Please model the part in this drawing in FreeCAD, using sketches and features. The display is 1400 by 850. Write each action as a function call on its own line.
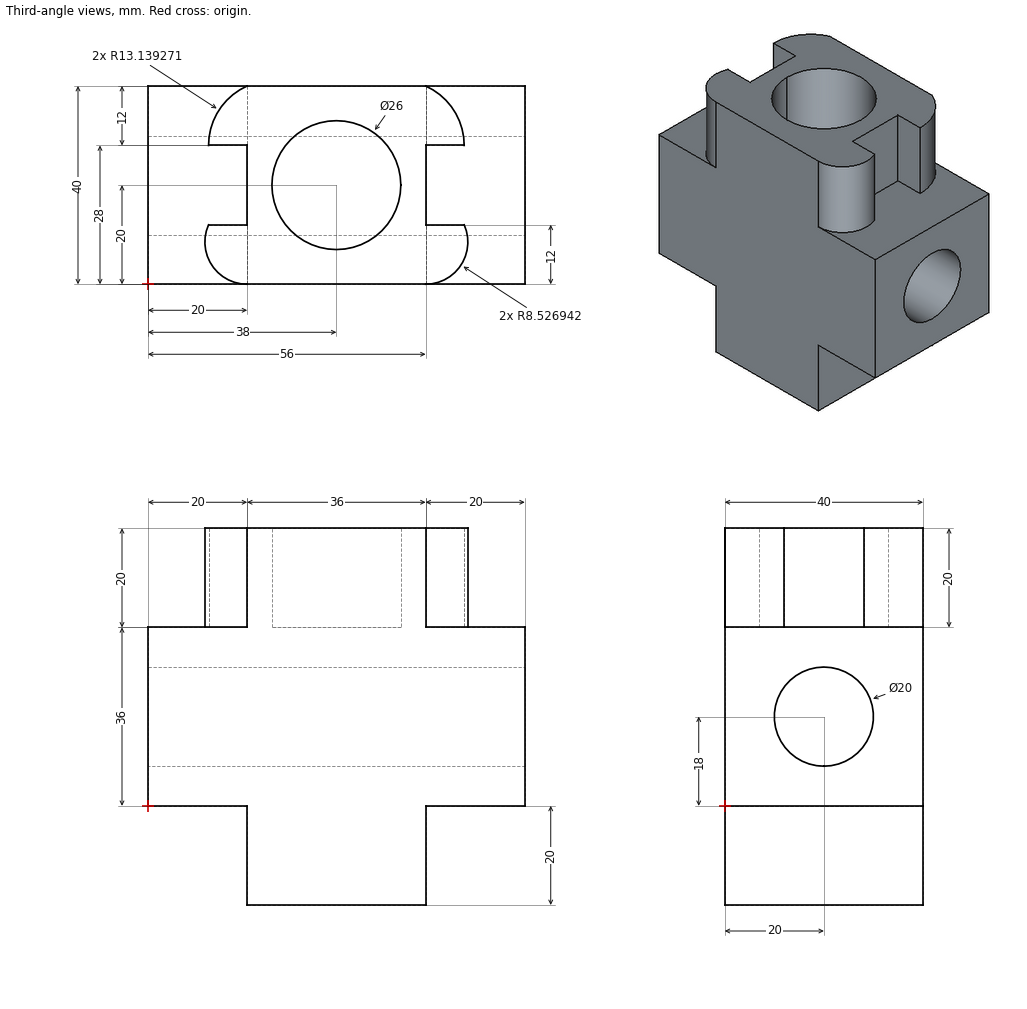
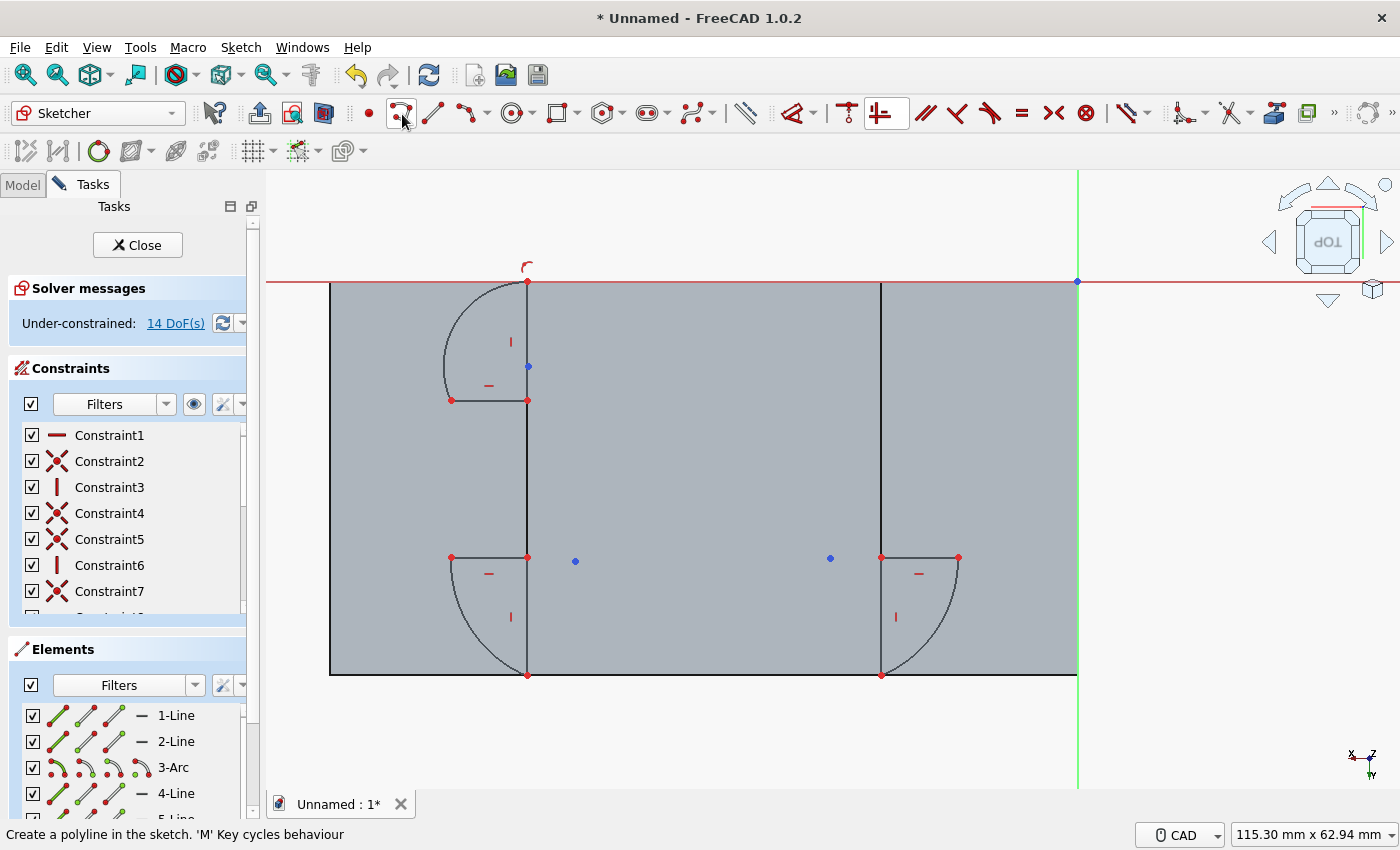
click(881, 282)
click(881, 400)
click(958, 400)
right_click(958, 400)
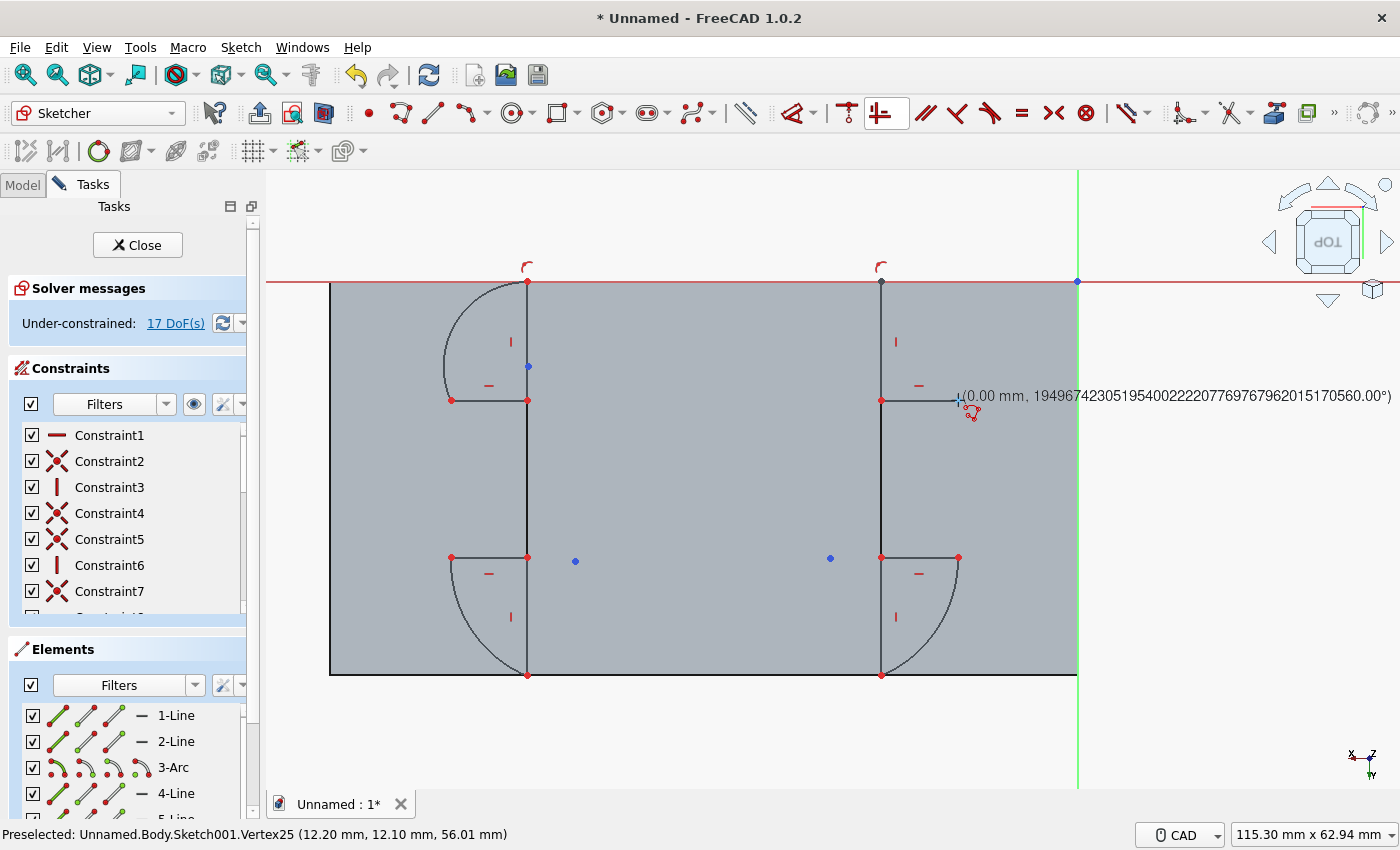
click(466, 114)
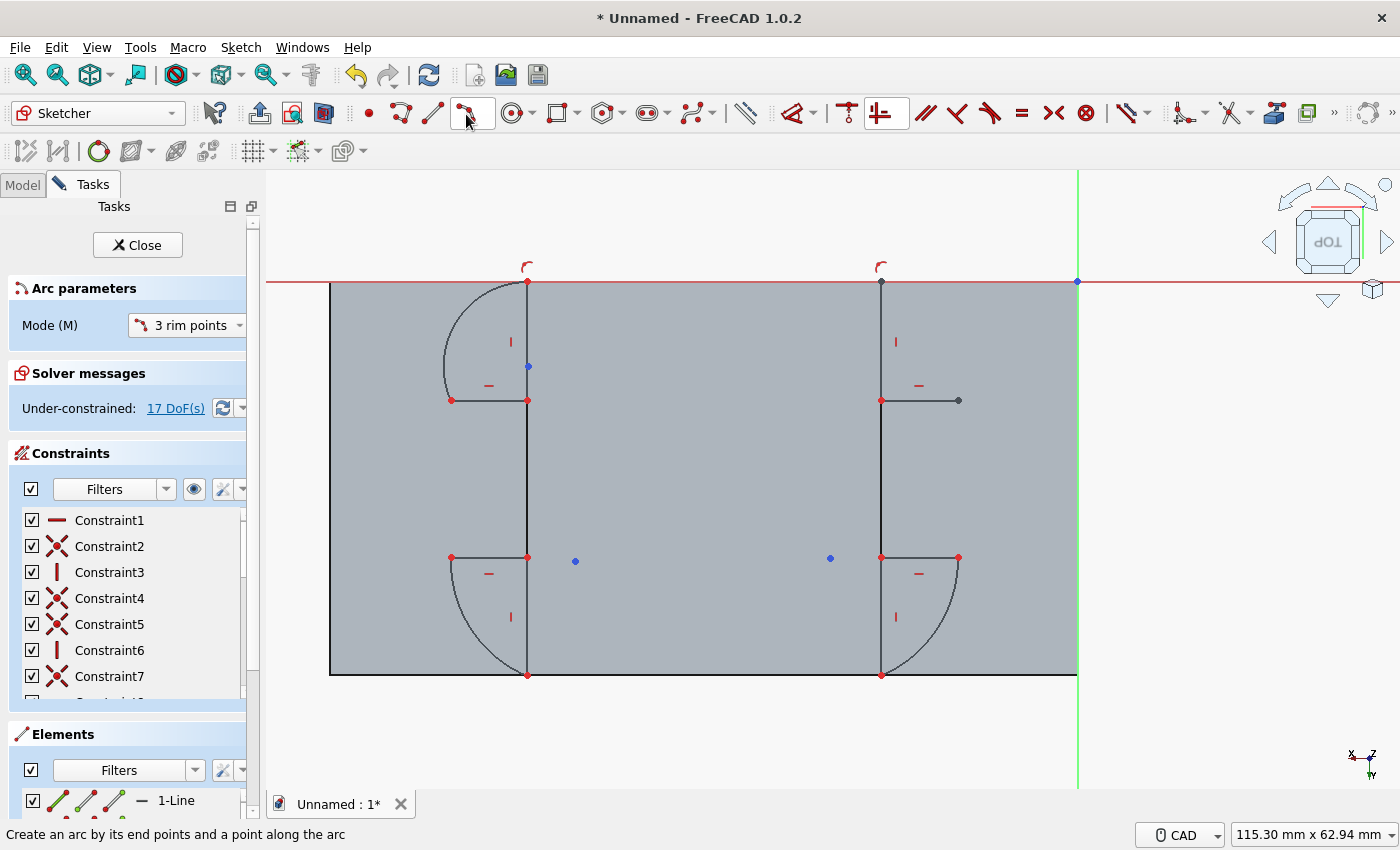
click(958, 401)
click(881, 282)
click(952, 320)
key(Escape)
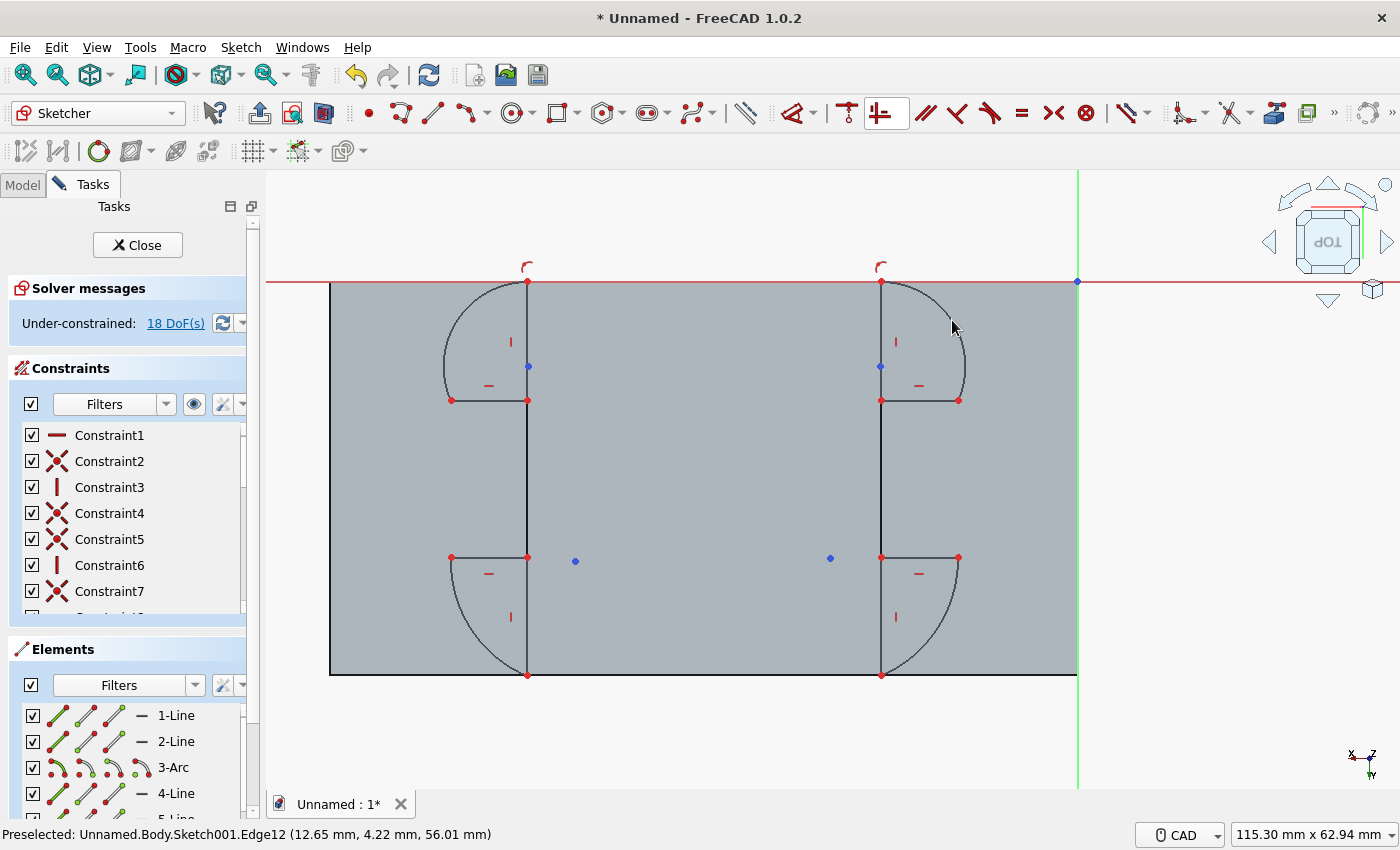
click(918, 651)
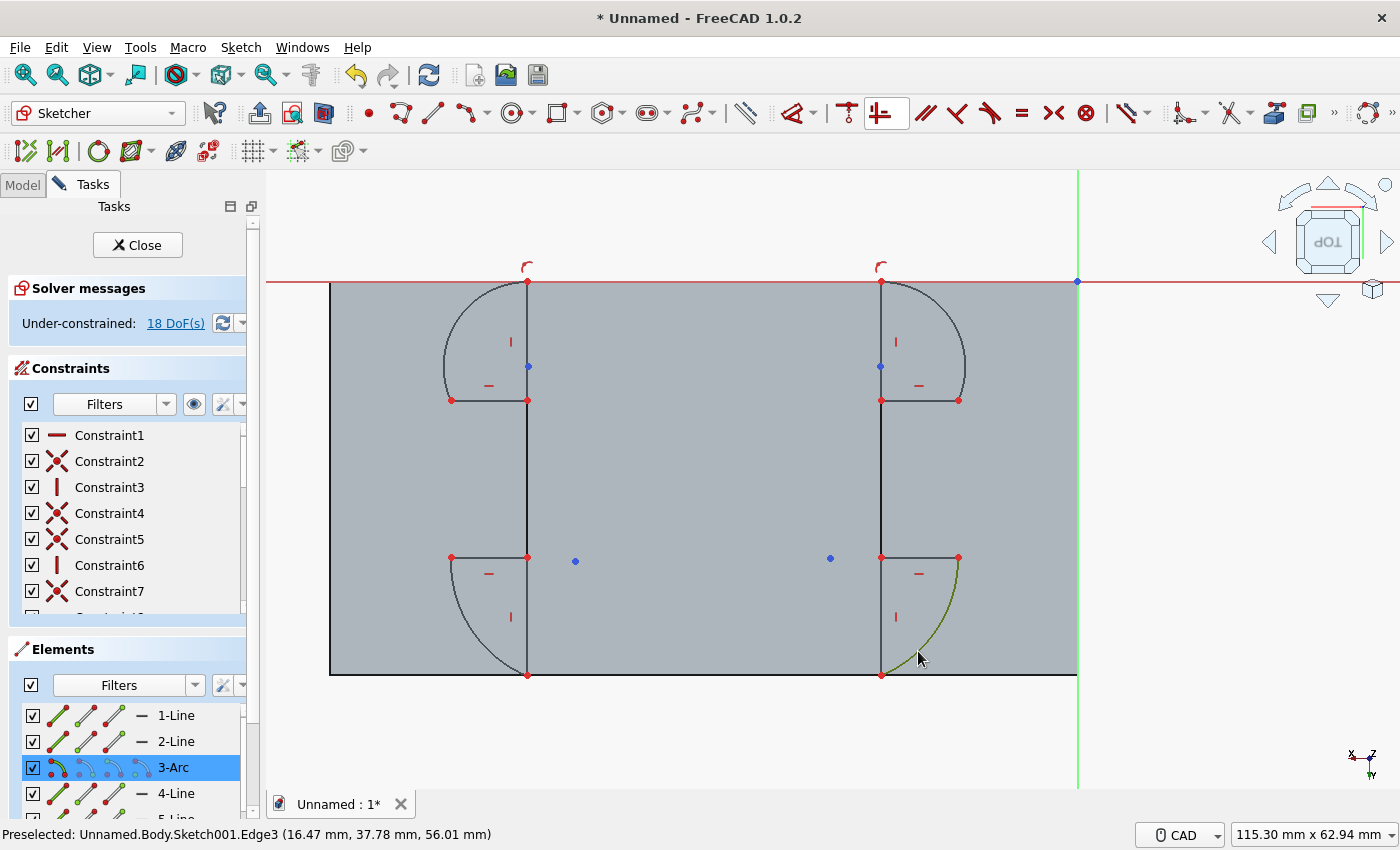
click(458, 602)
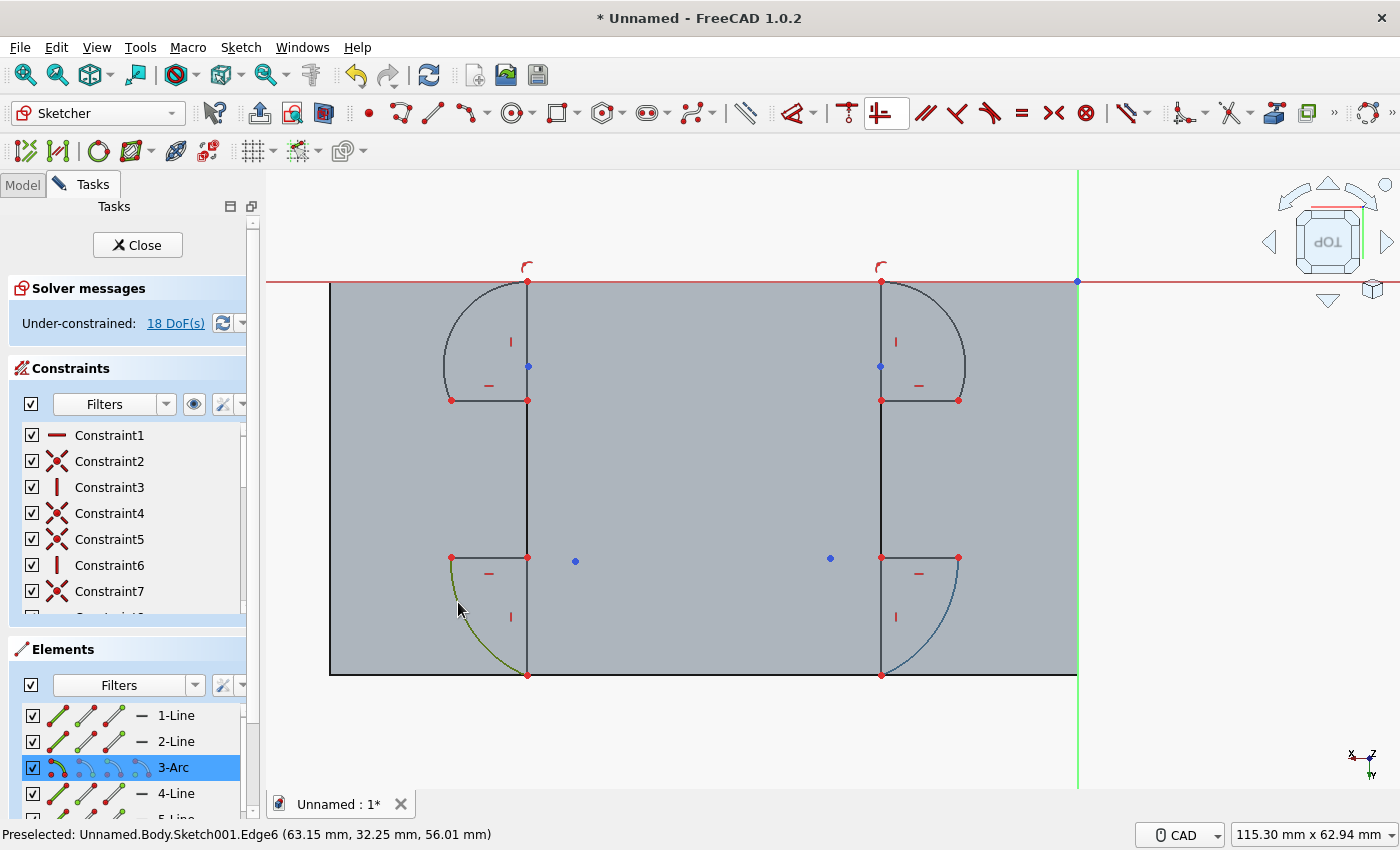
click(1022, 114)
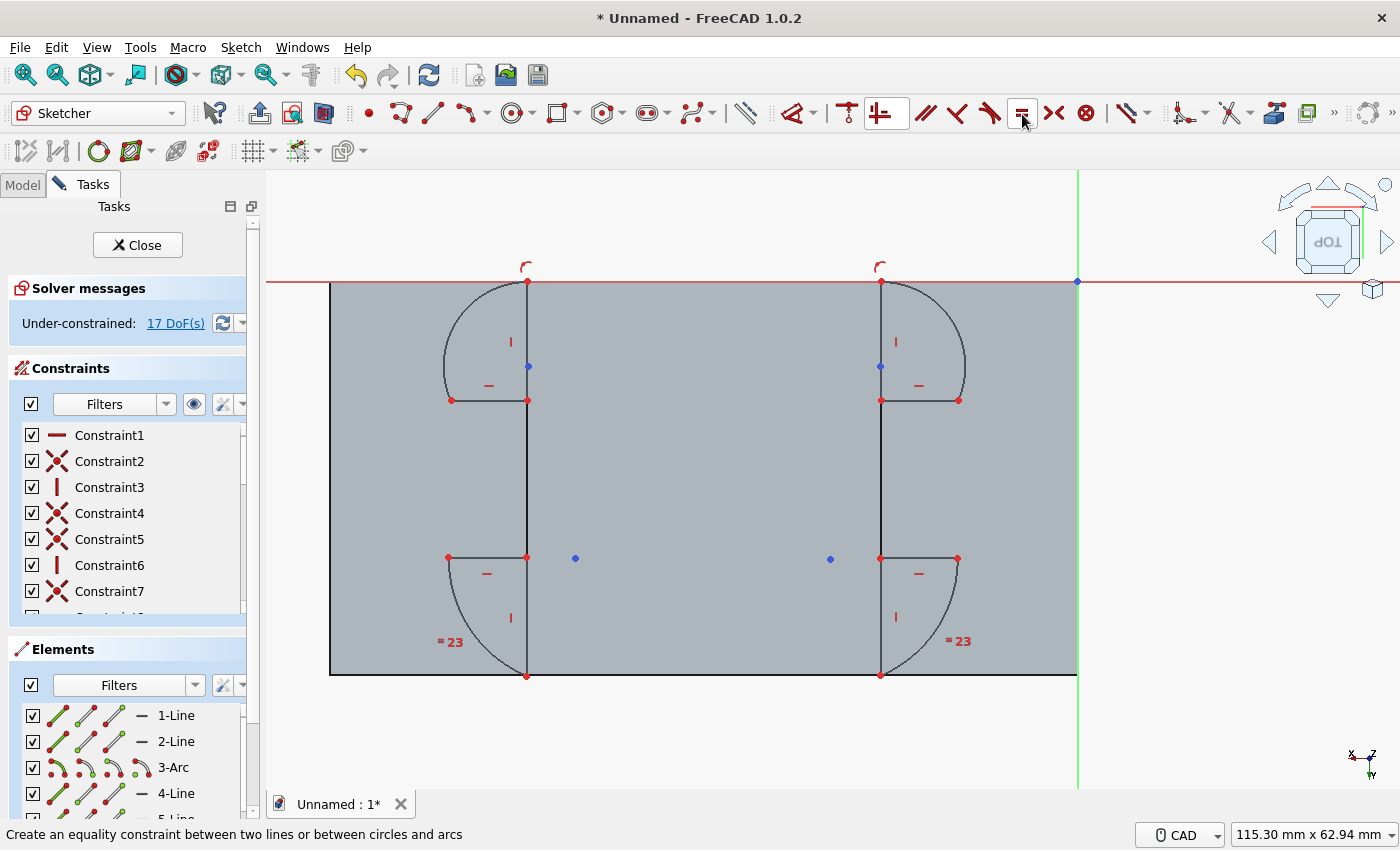
click(480, 297)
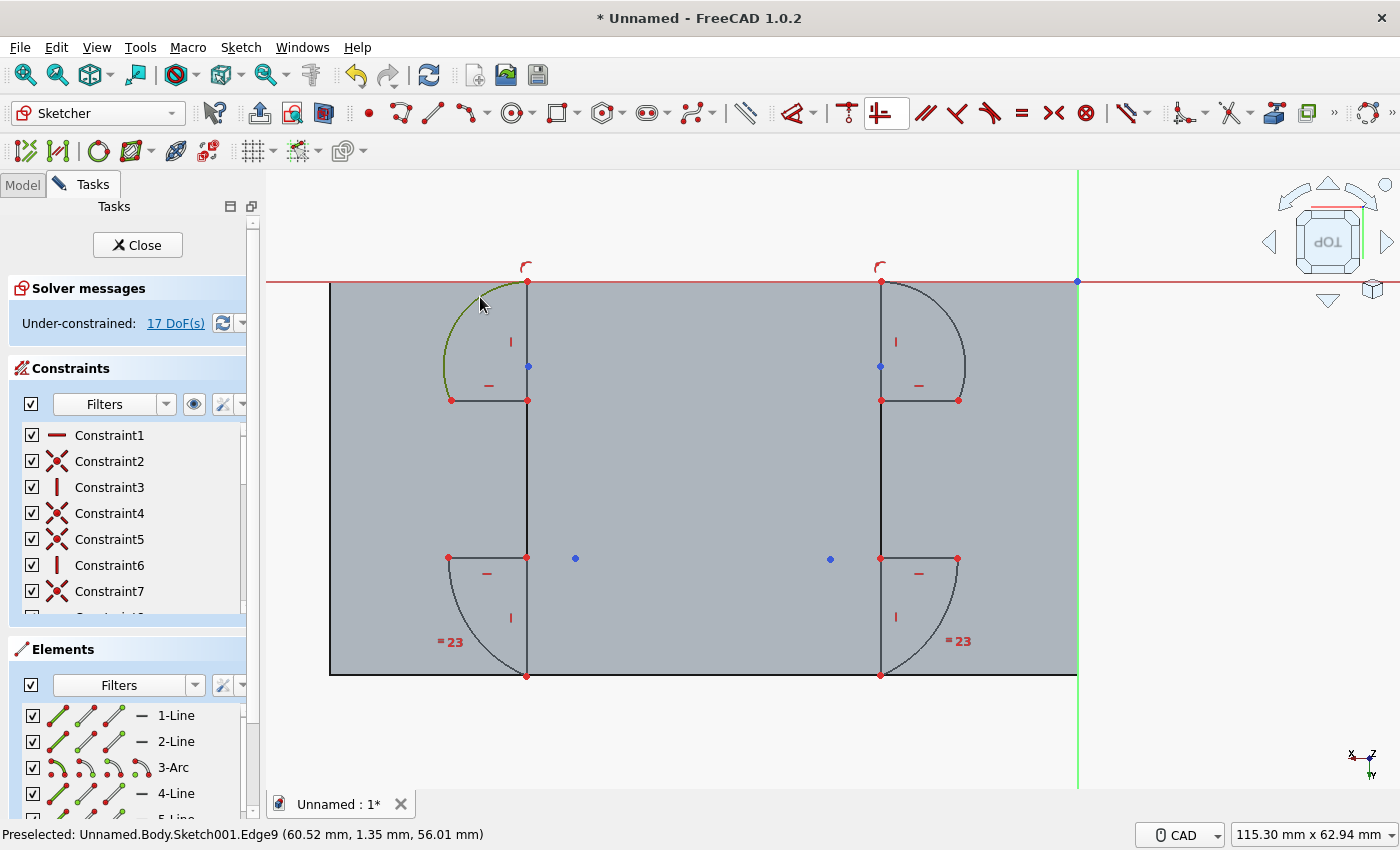
click(964, 352)